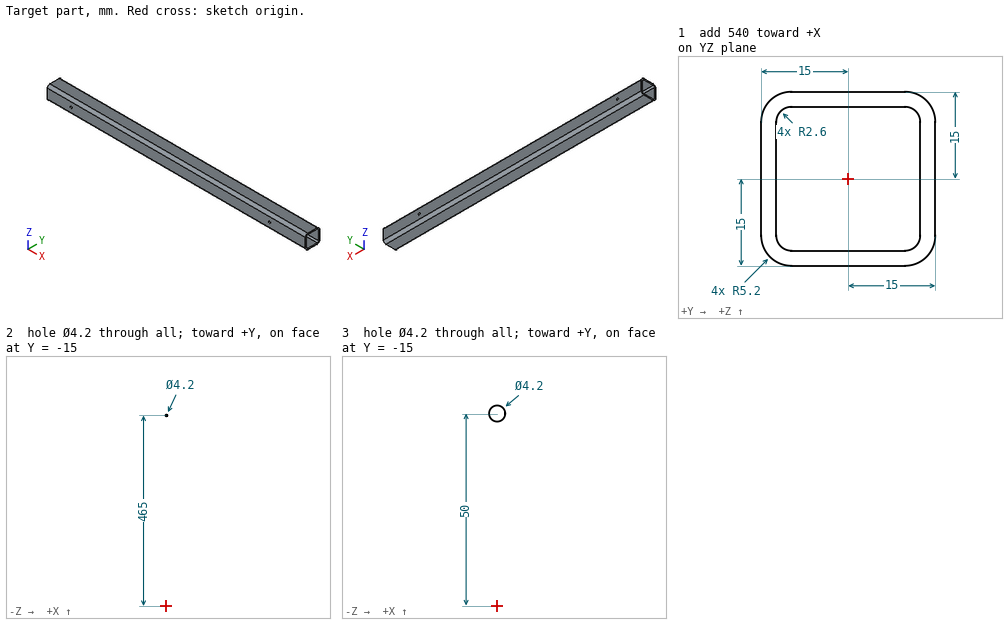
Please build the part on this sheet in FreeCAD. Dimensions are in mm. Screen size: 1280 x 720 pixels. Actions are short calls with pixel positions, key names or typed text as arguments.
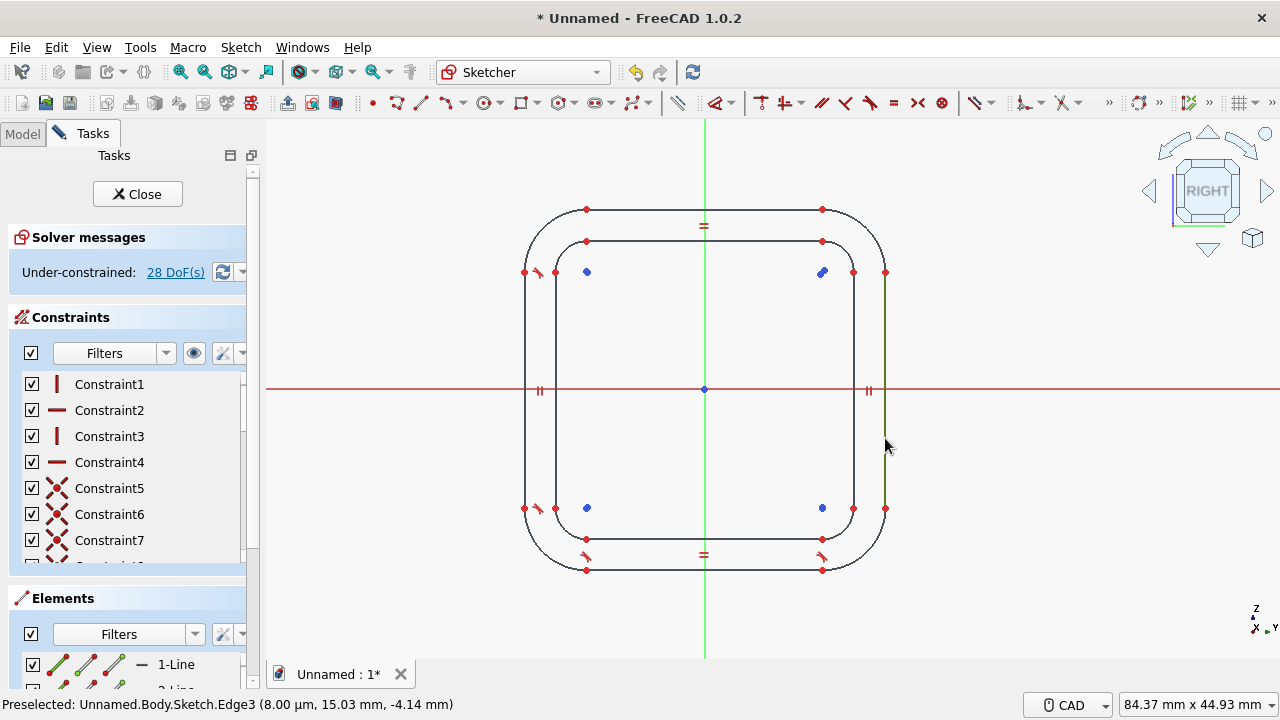
click(851, 564)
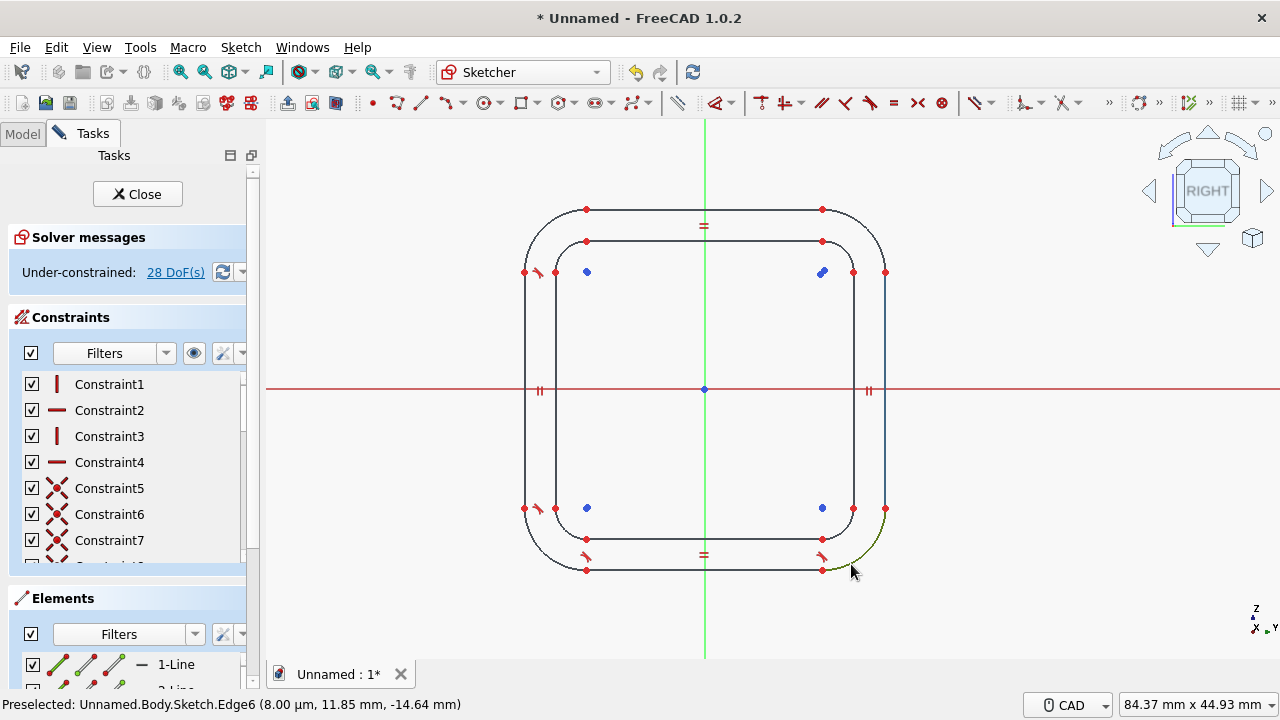
click(870, 104)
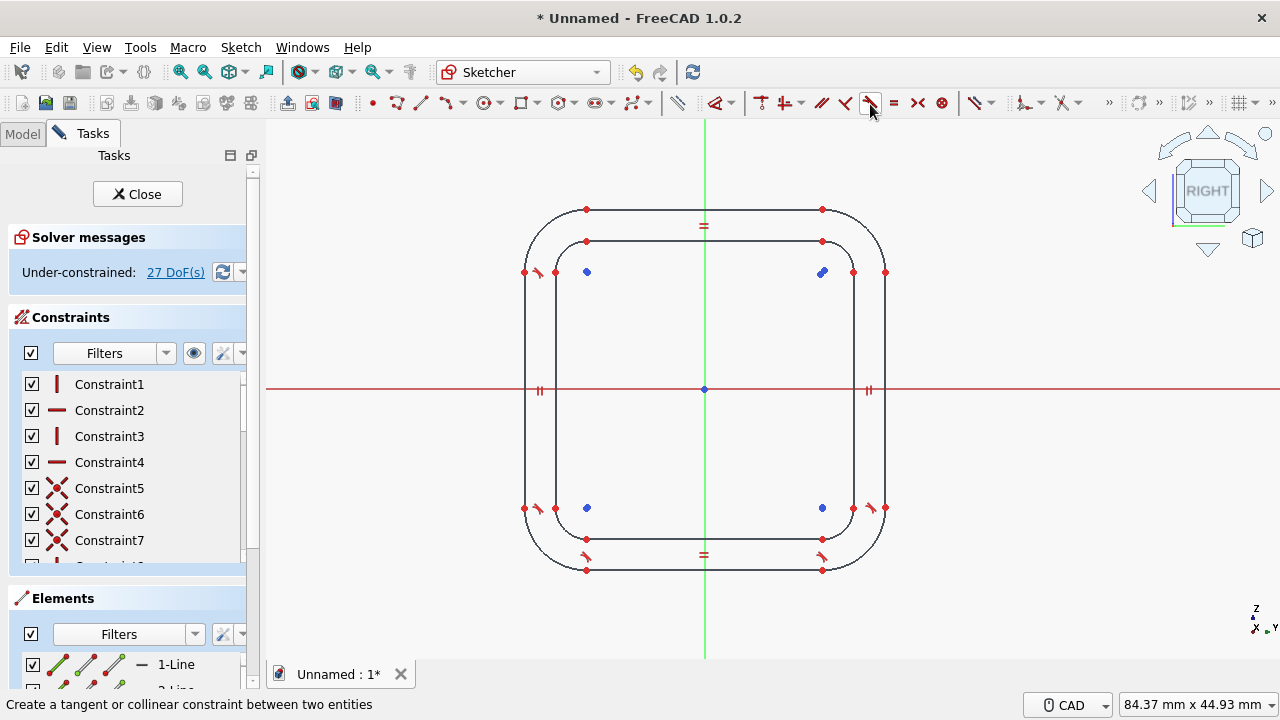
click(885, 437)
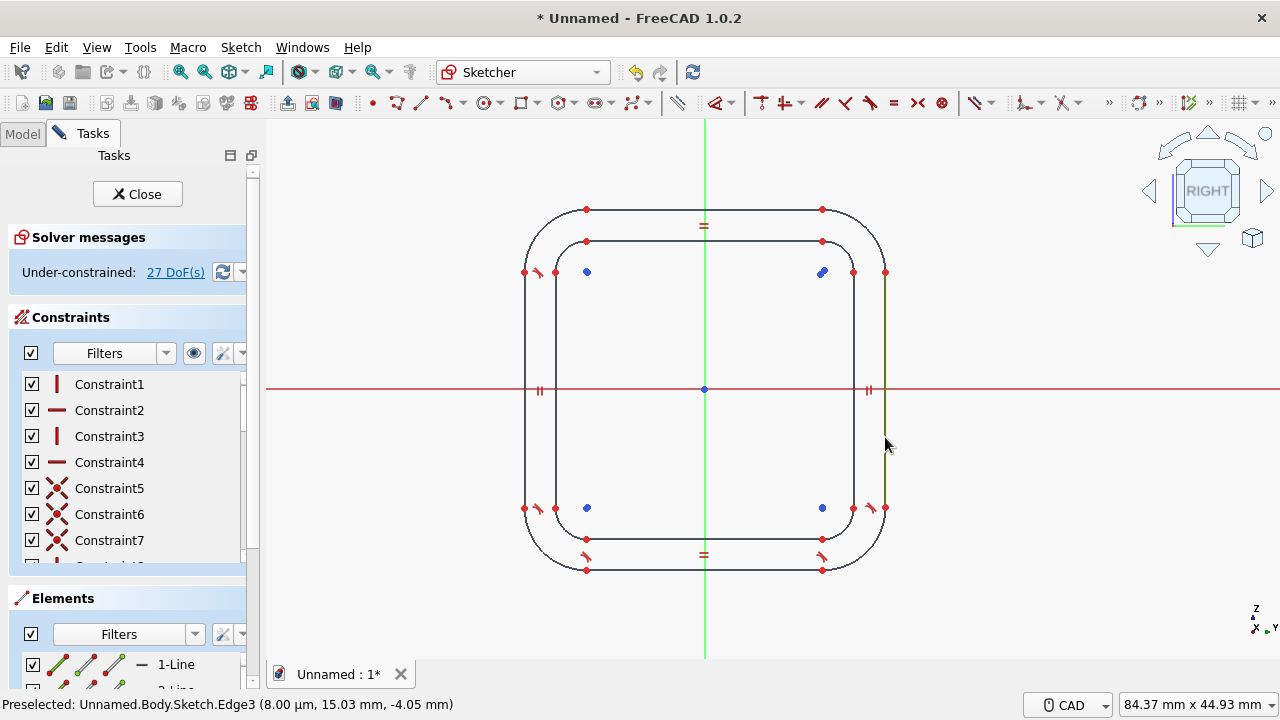
click(878, 244)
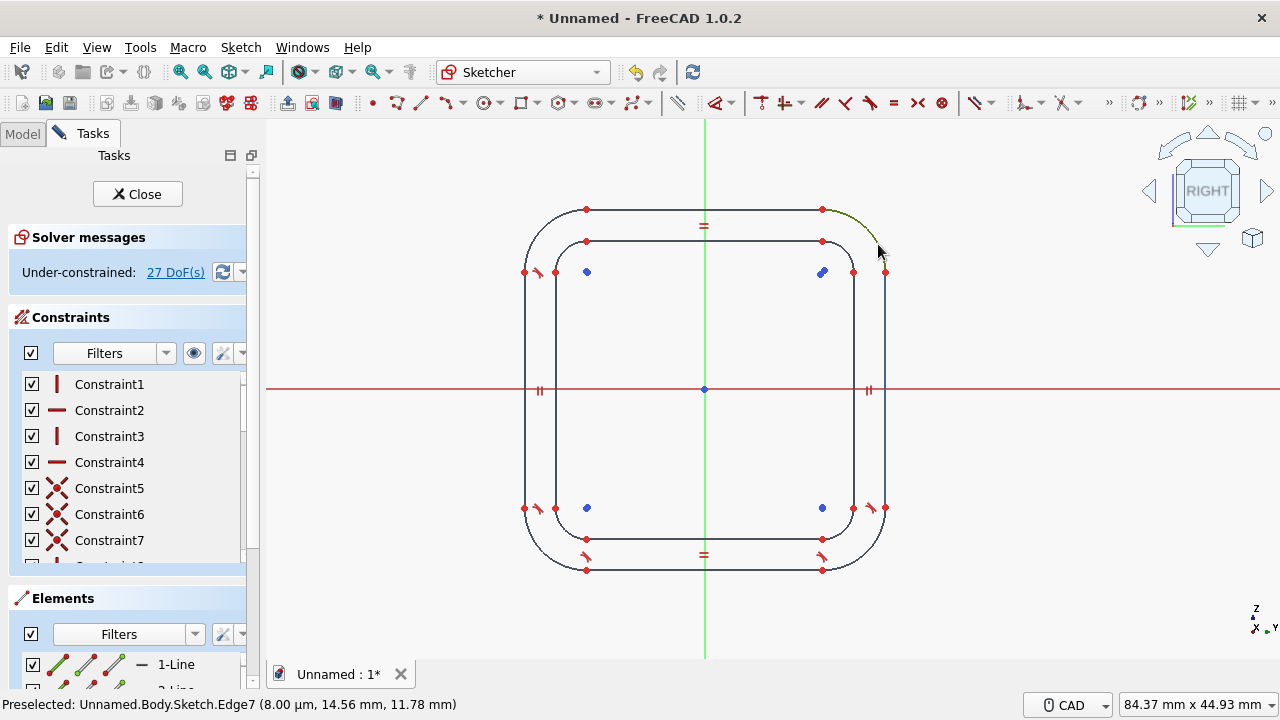
key(t)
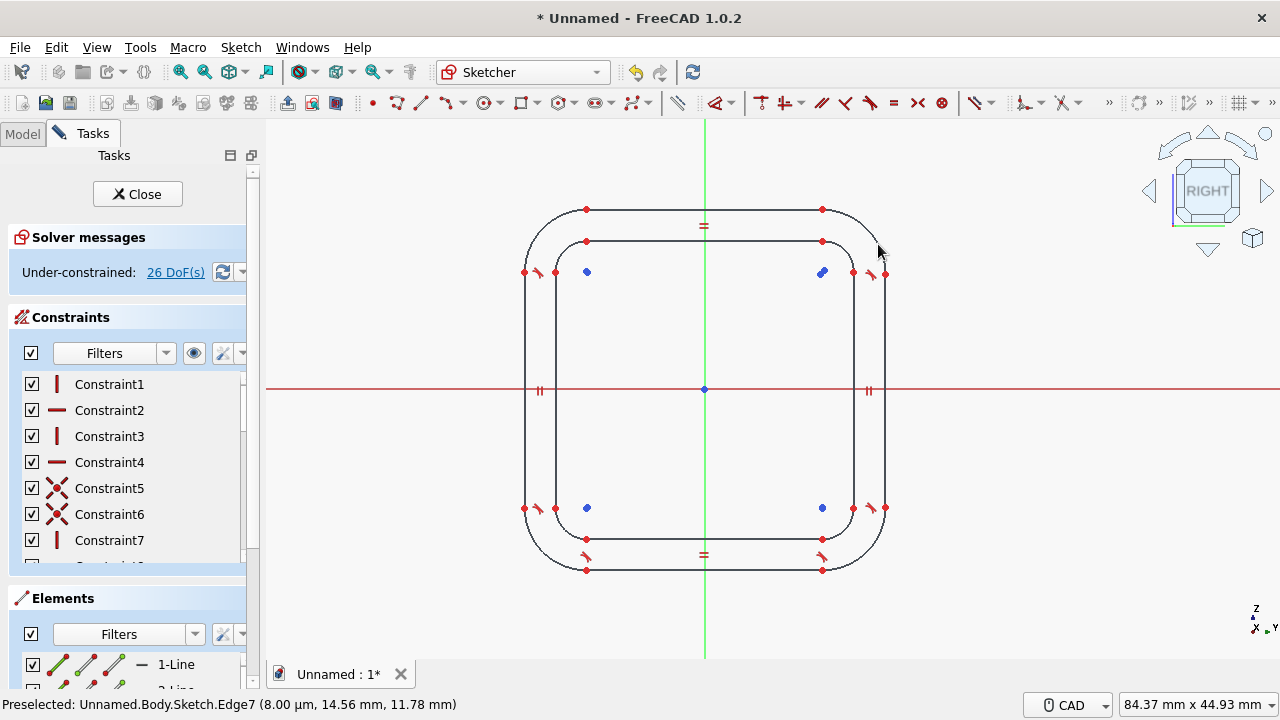
click(752, 210)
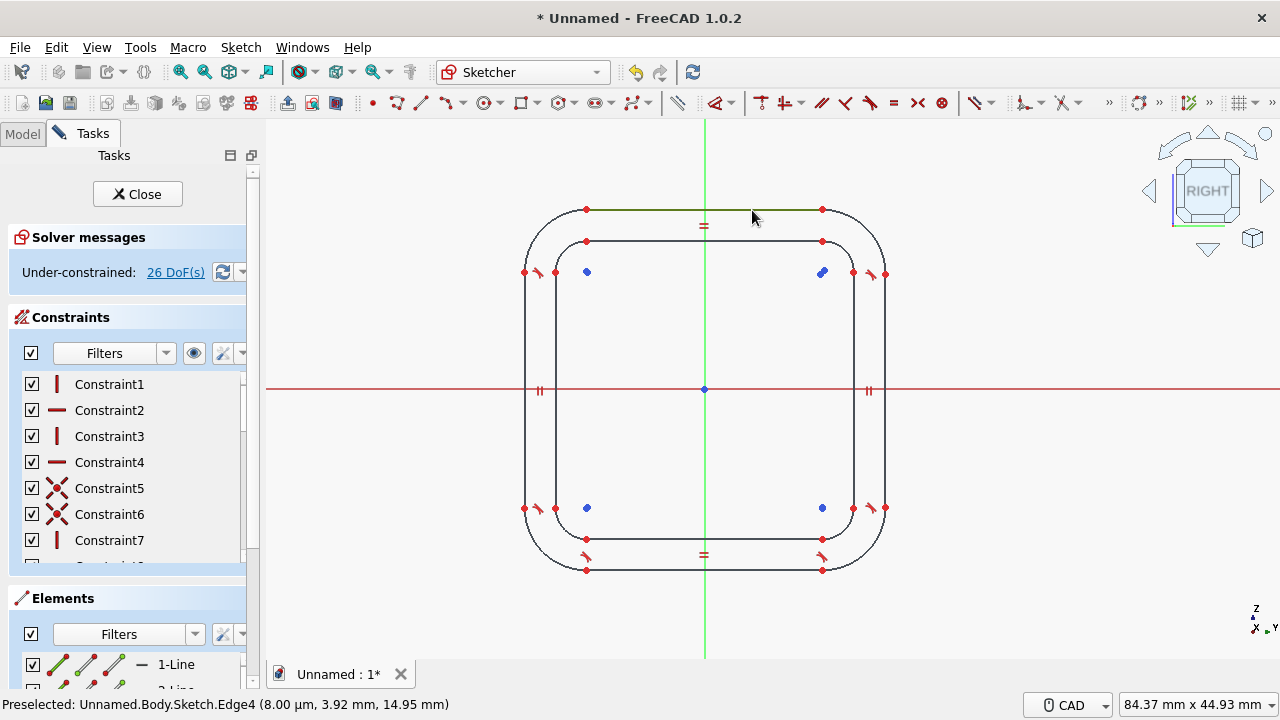
click(879, 245)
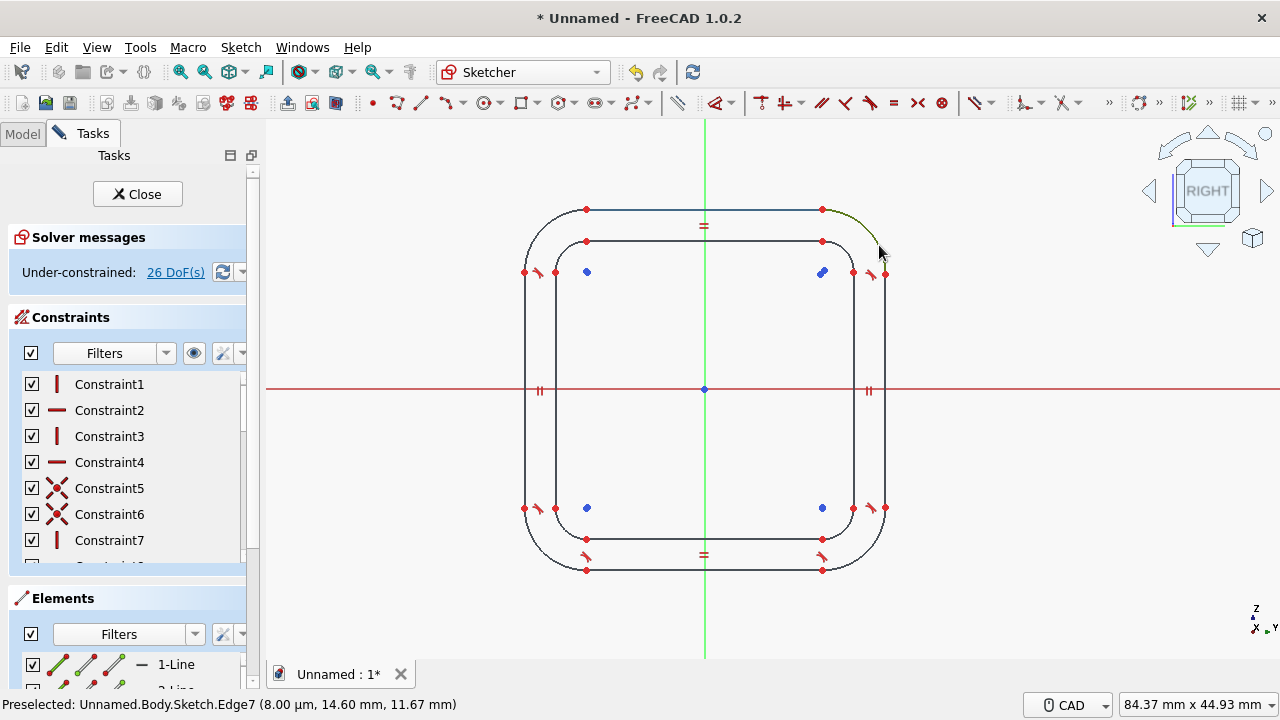
click(870, 104)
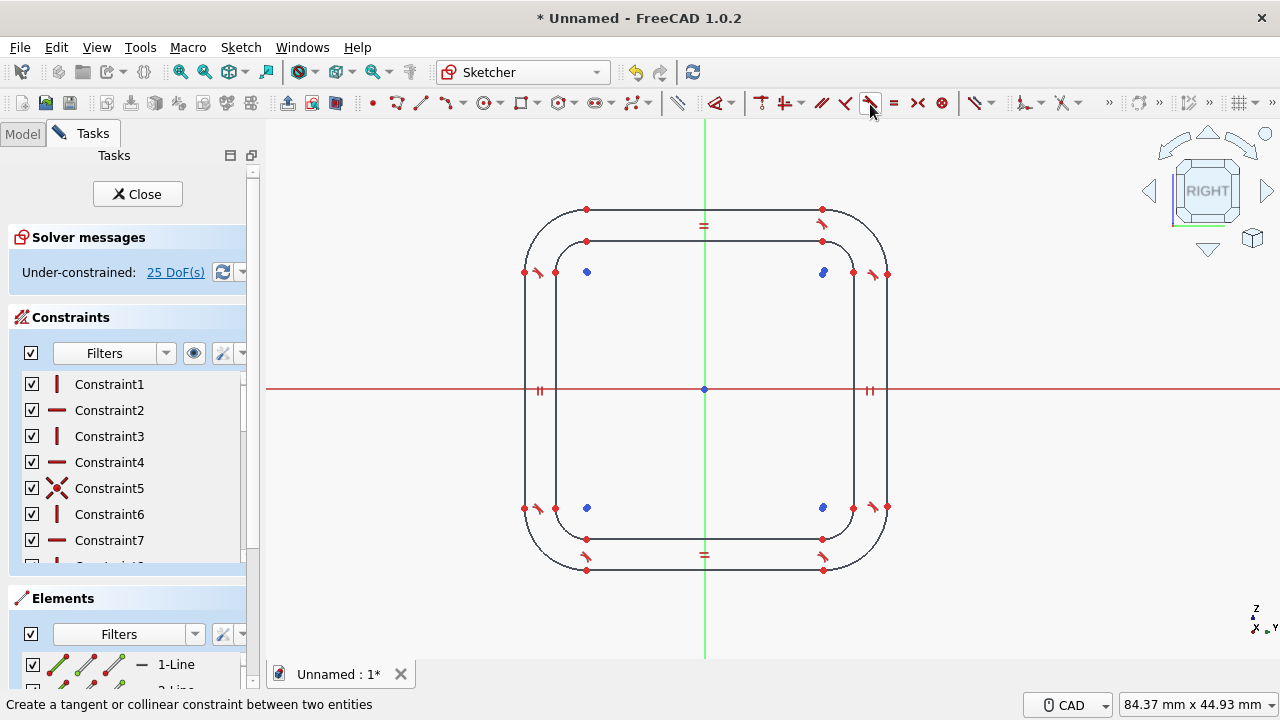
click(752, 210)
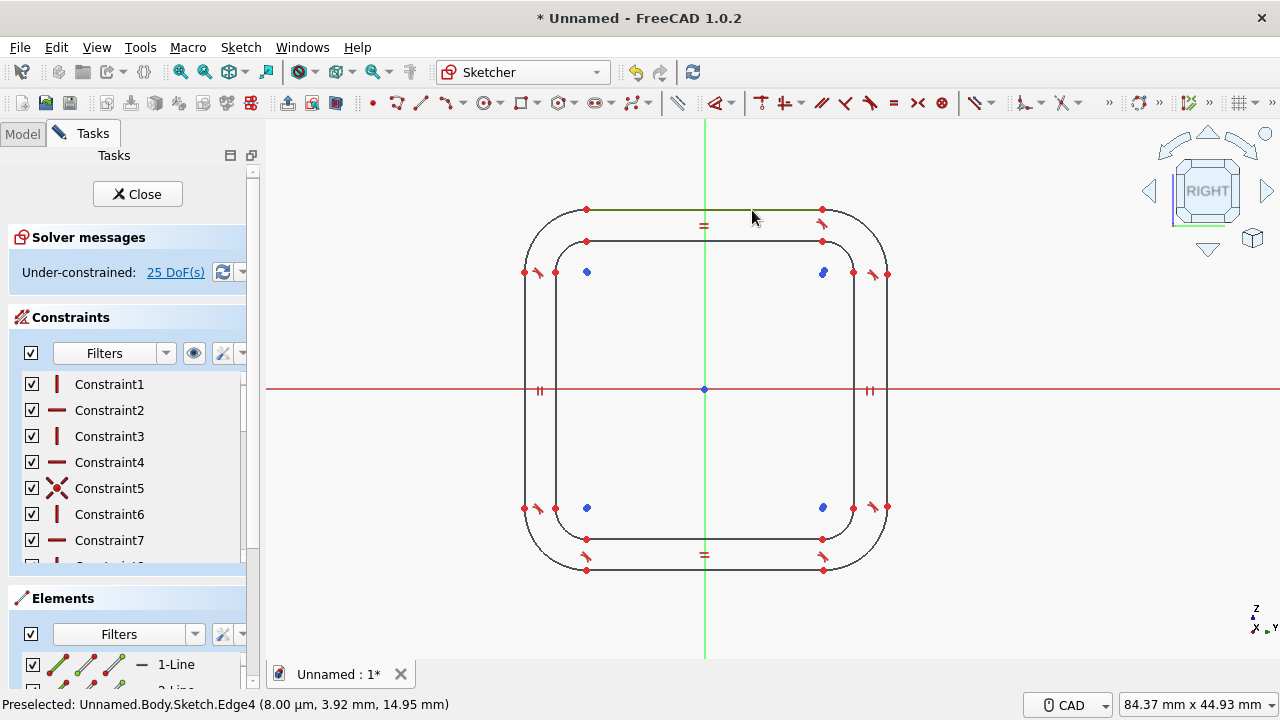
click(558, 217)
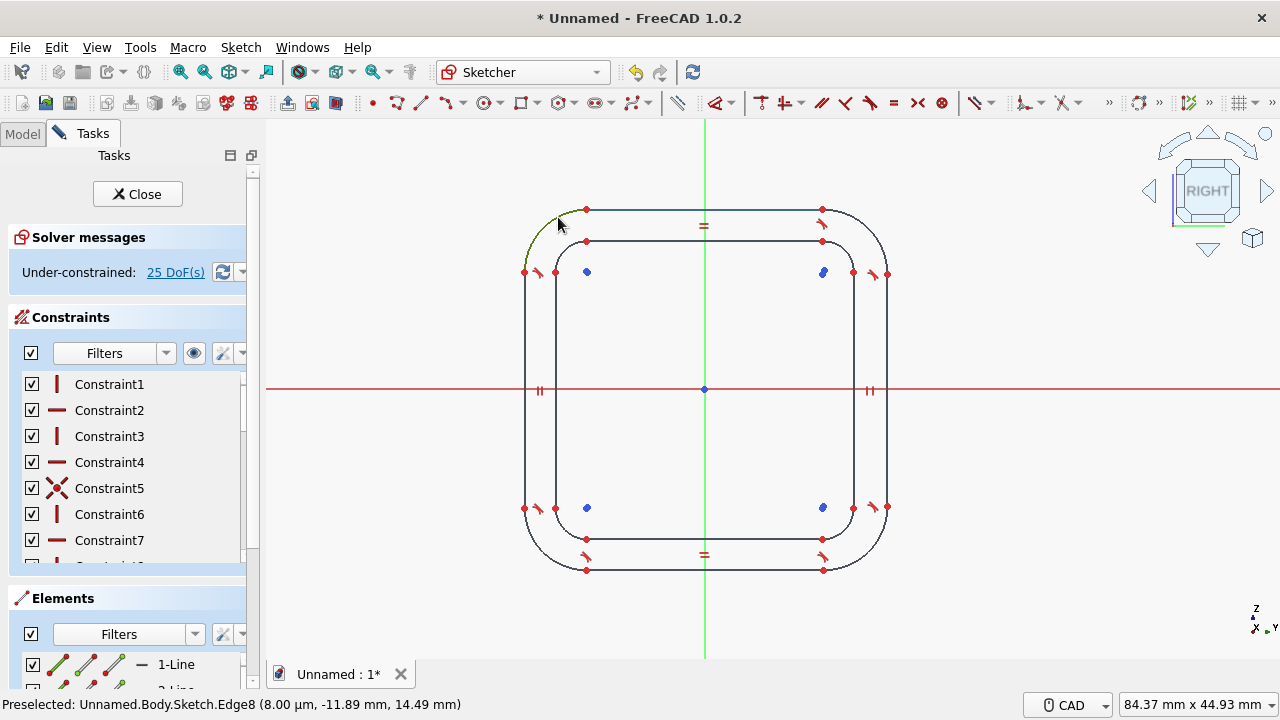
key(t)